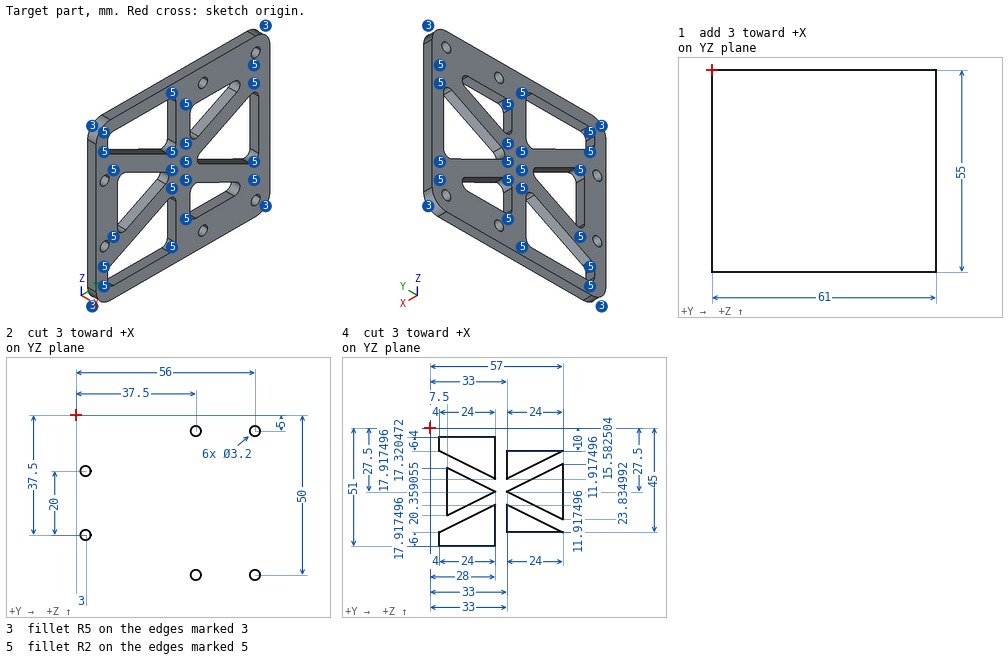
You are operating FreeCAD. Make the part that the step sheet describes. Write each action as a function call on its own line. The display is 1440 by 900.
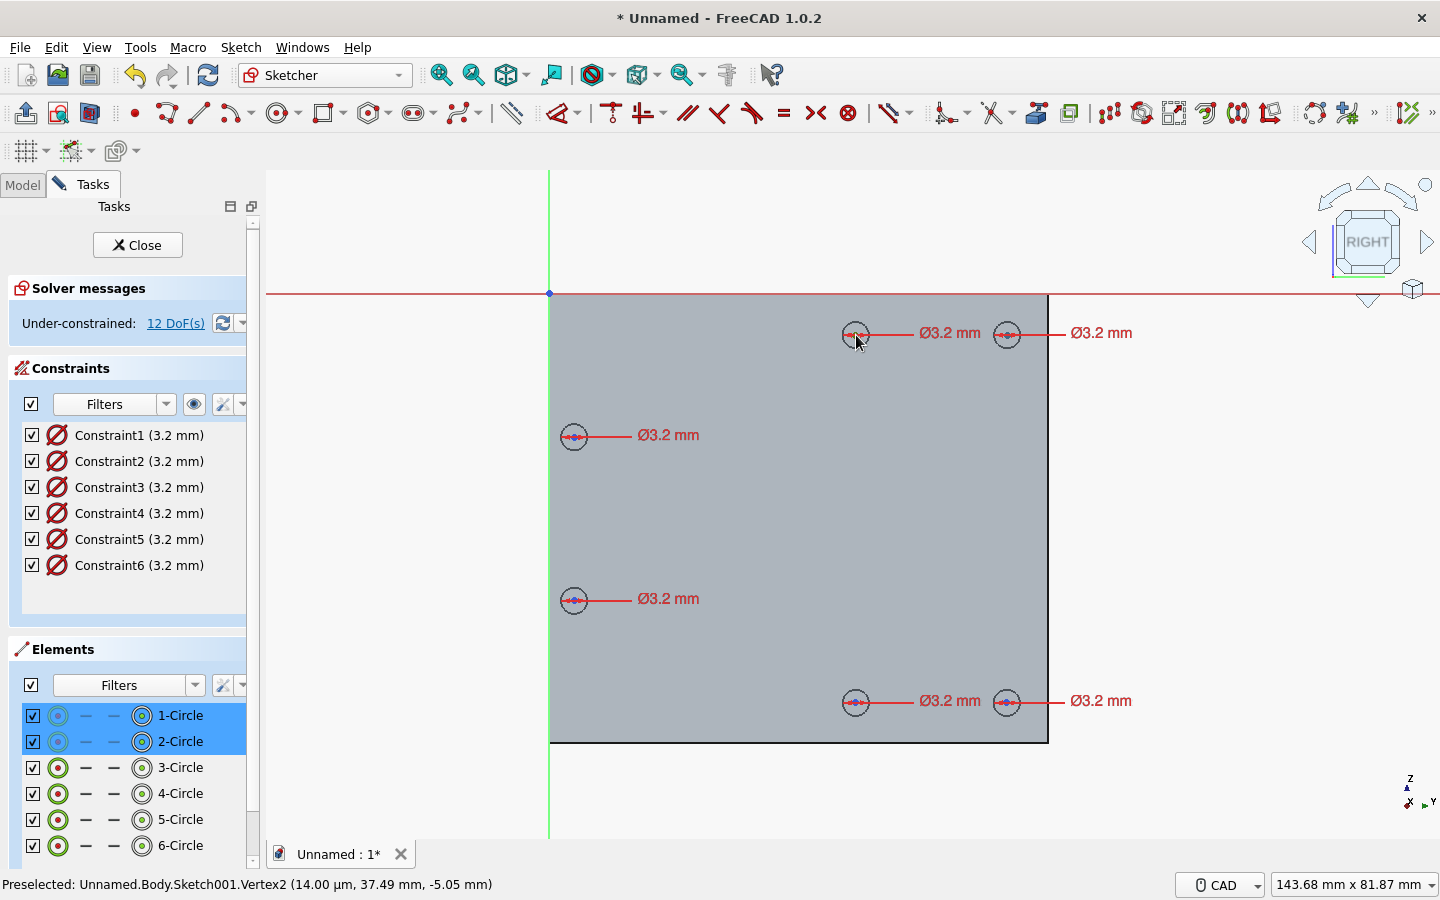
key(h)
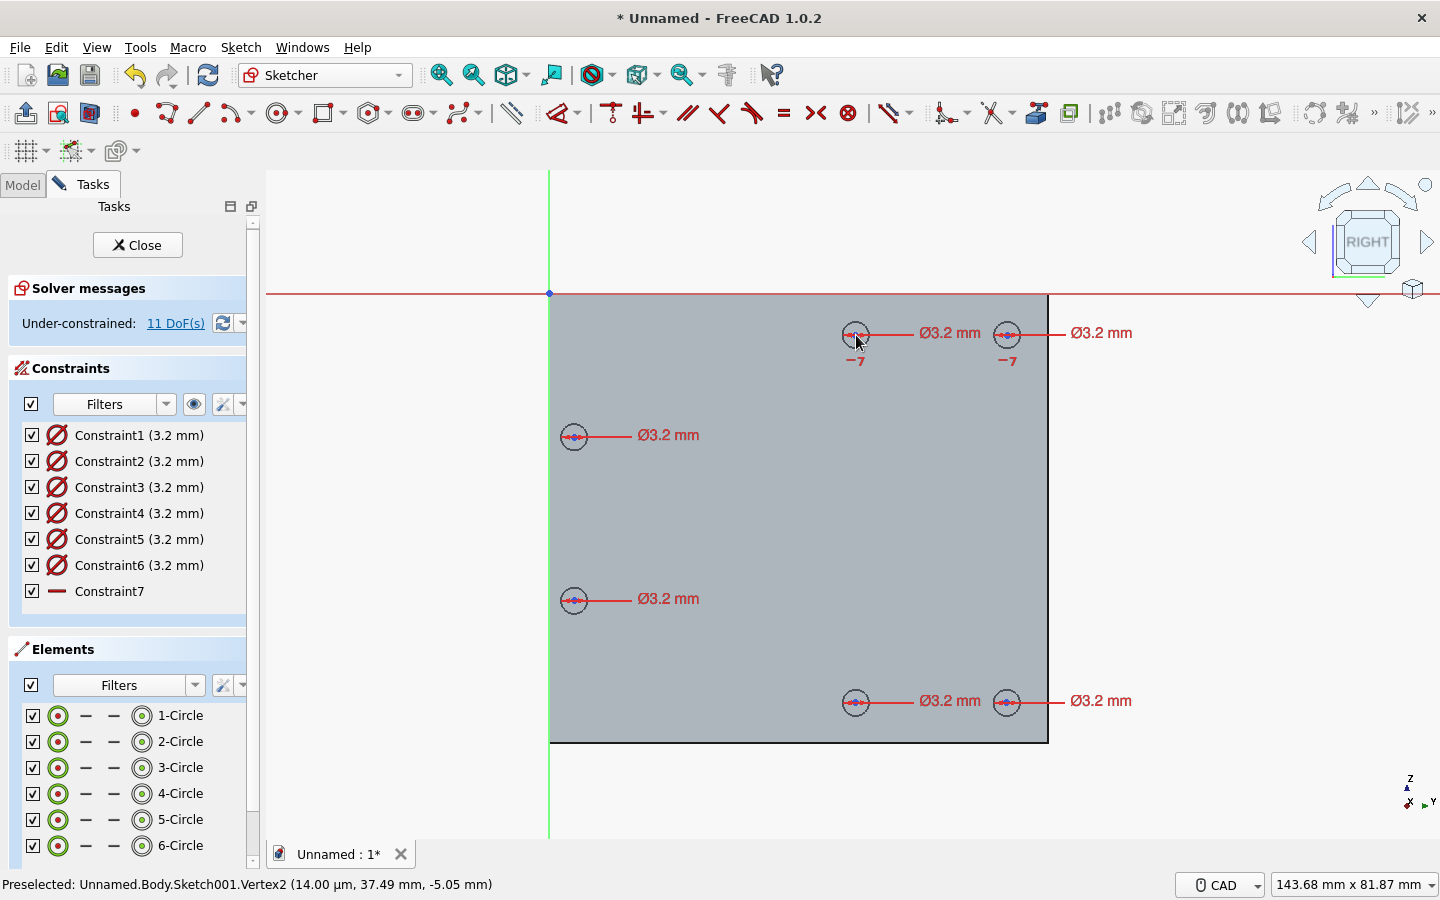
click(1007, 335)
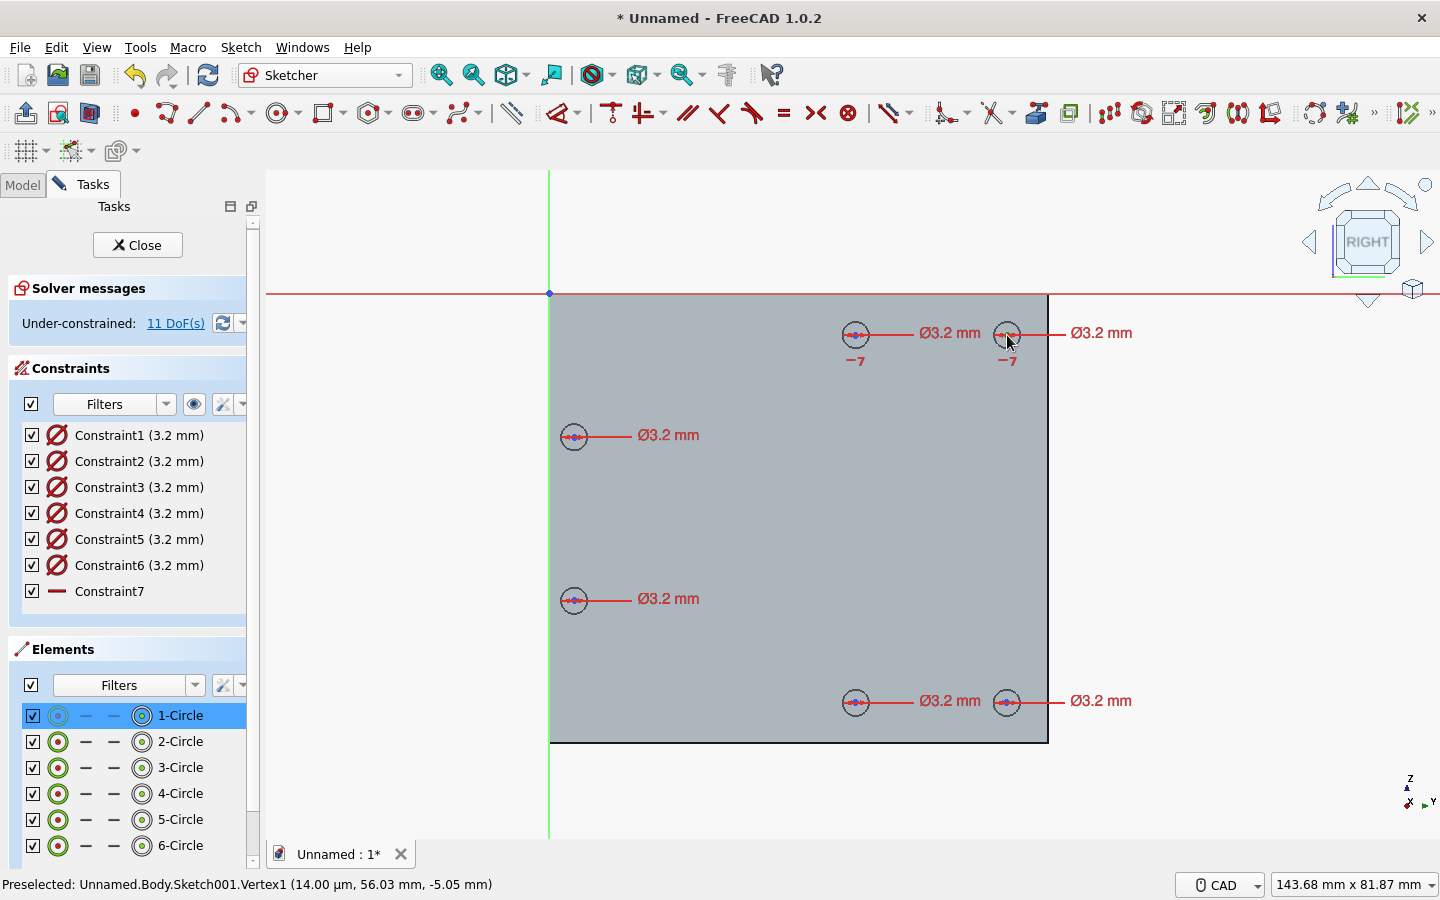
click(1007, 703)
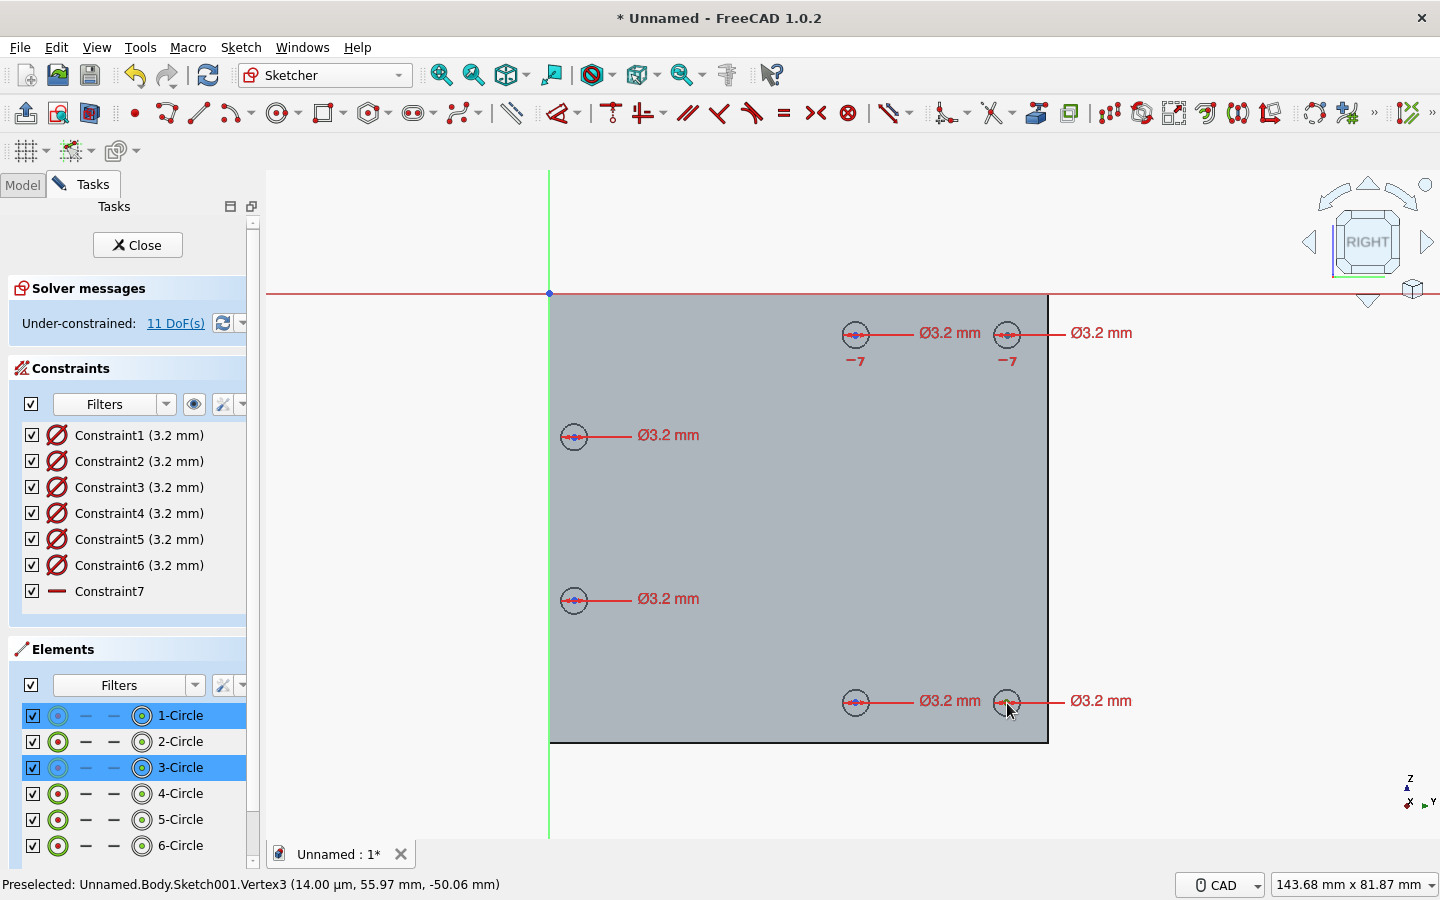
key(v)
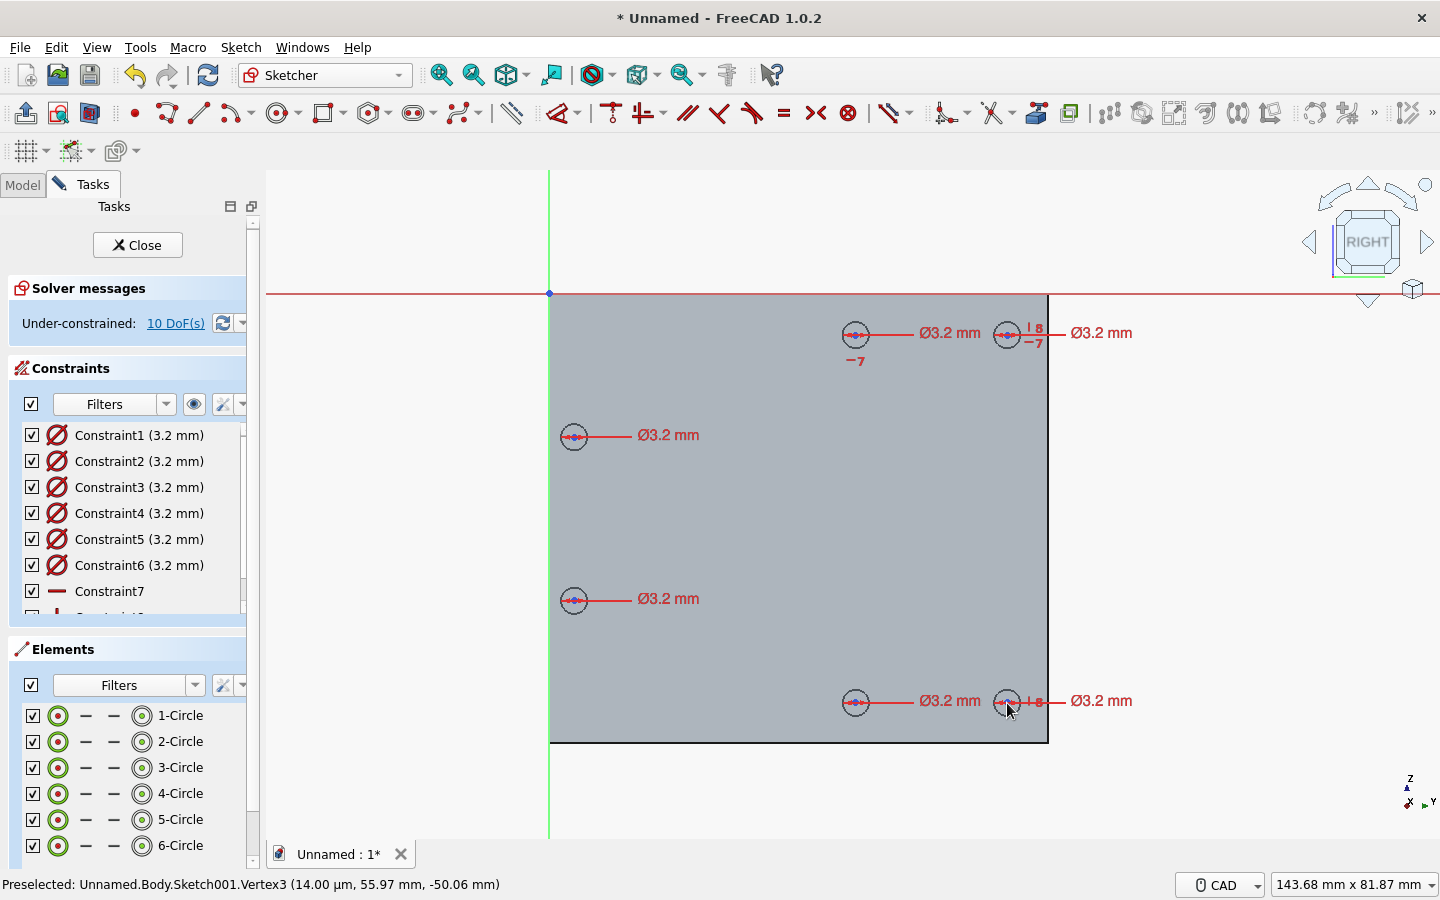
click(856, 335)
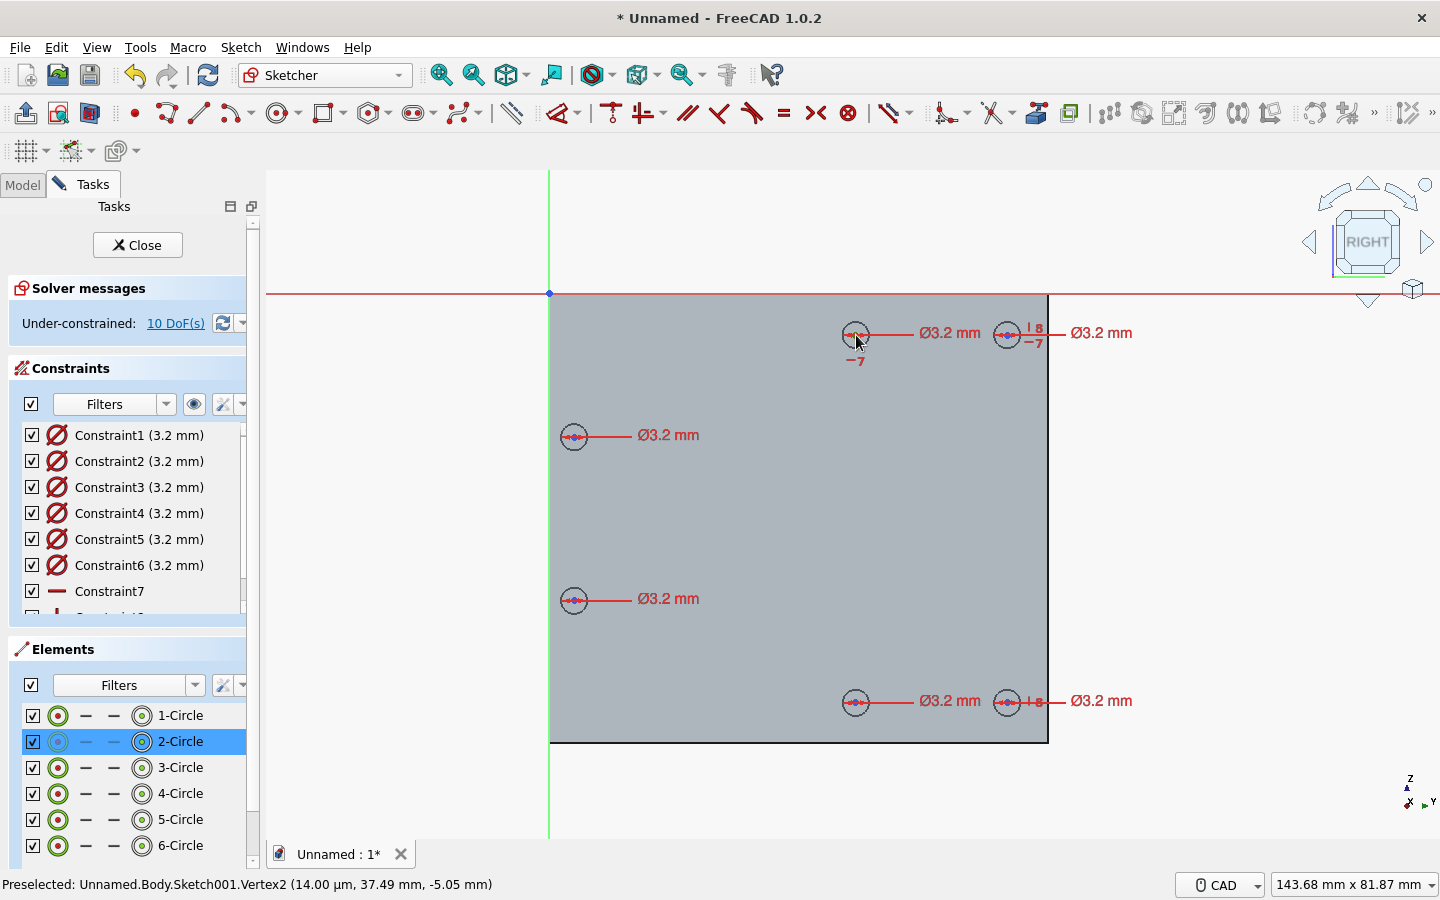
click(856, 703)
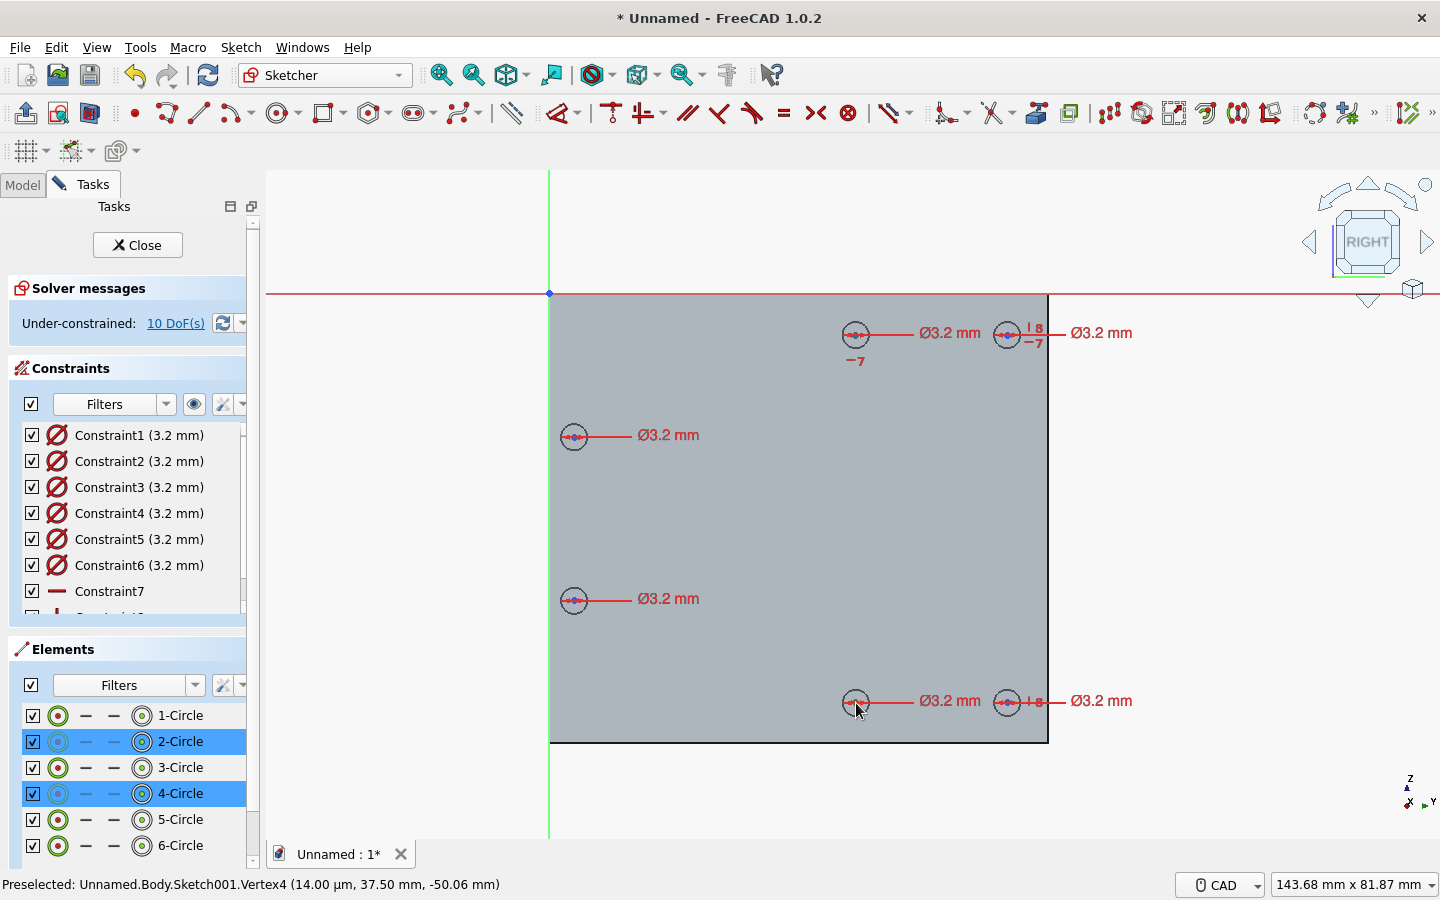
key(v)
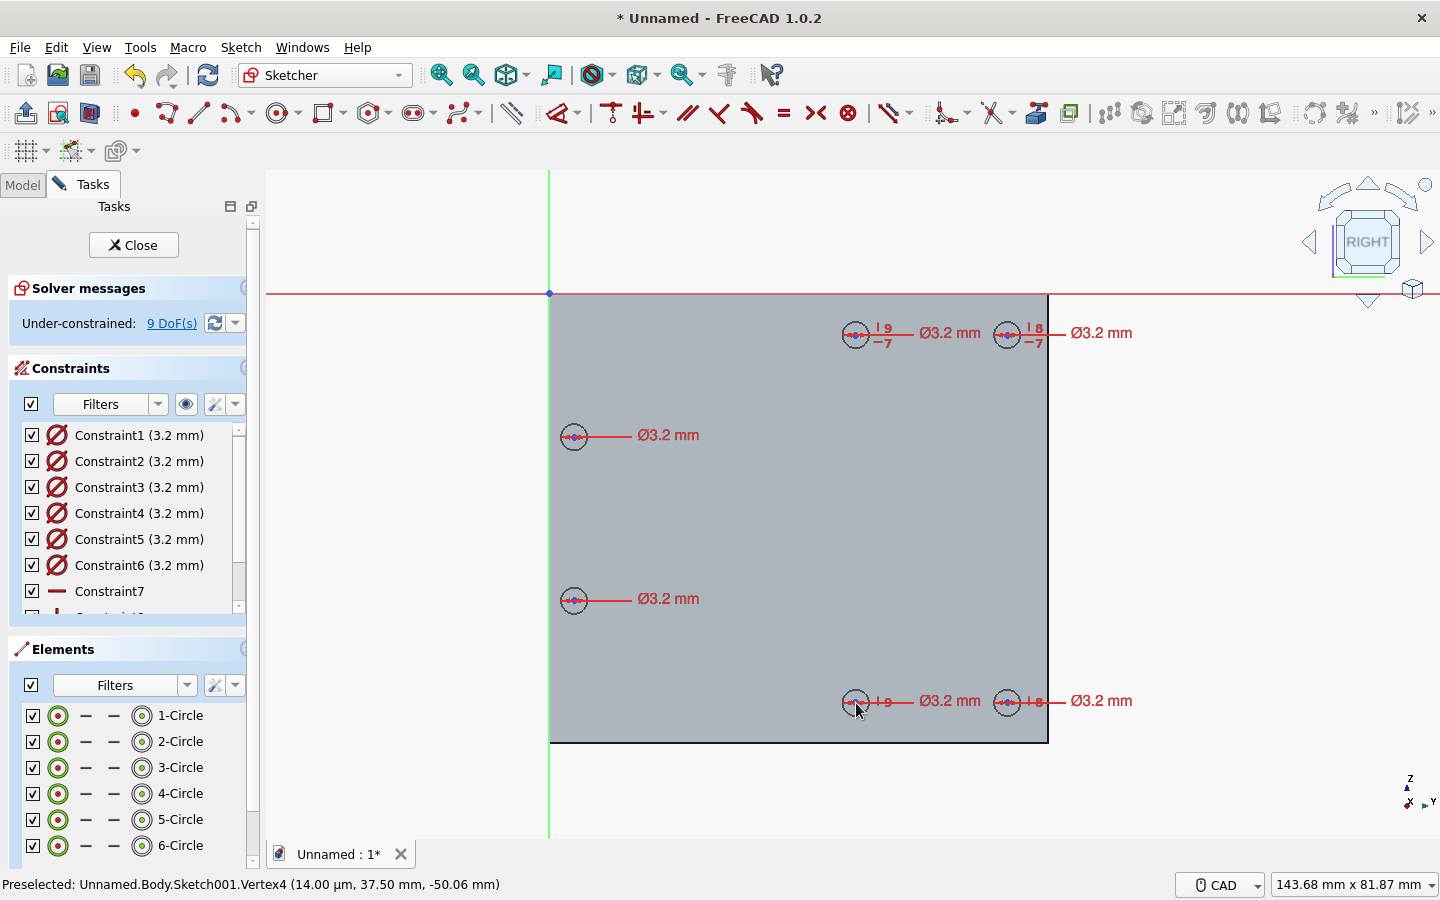
click(1007, 703)